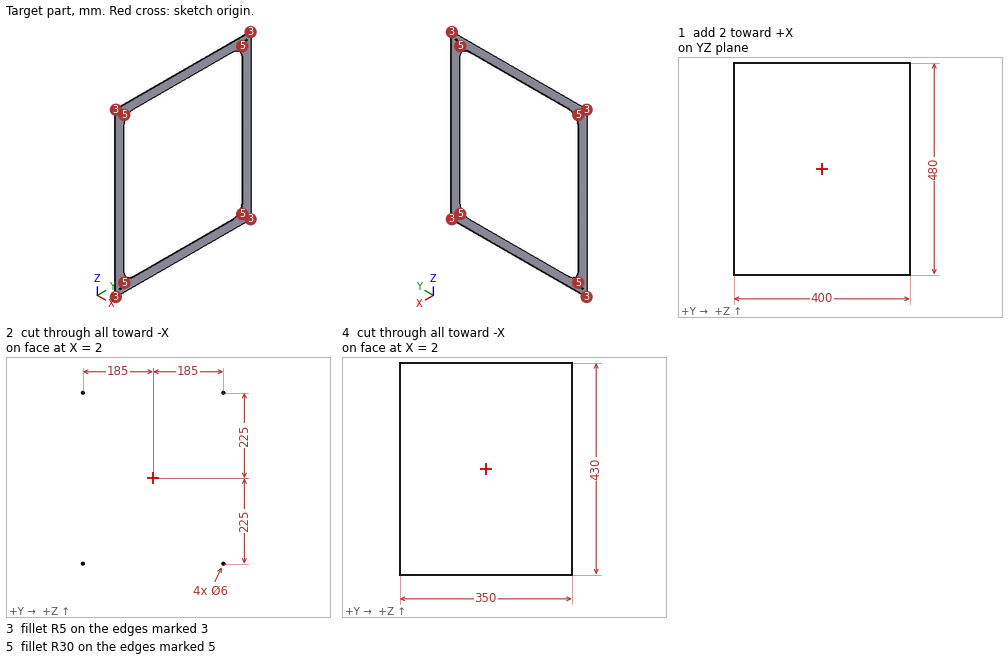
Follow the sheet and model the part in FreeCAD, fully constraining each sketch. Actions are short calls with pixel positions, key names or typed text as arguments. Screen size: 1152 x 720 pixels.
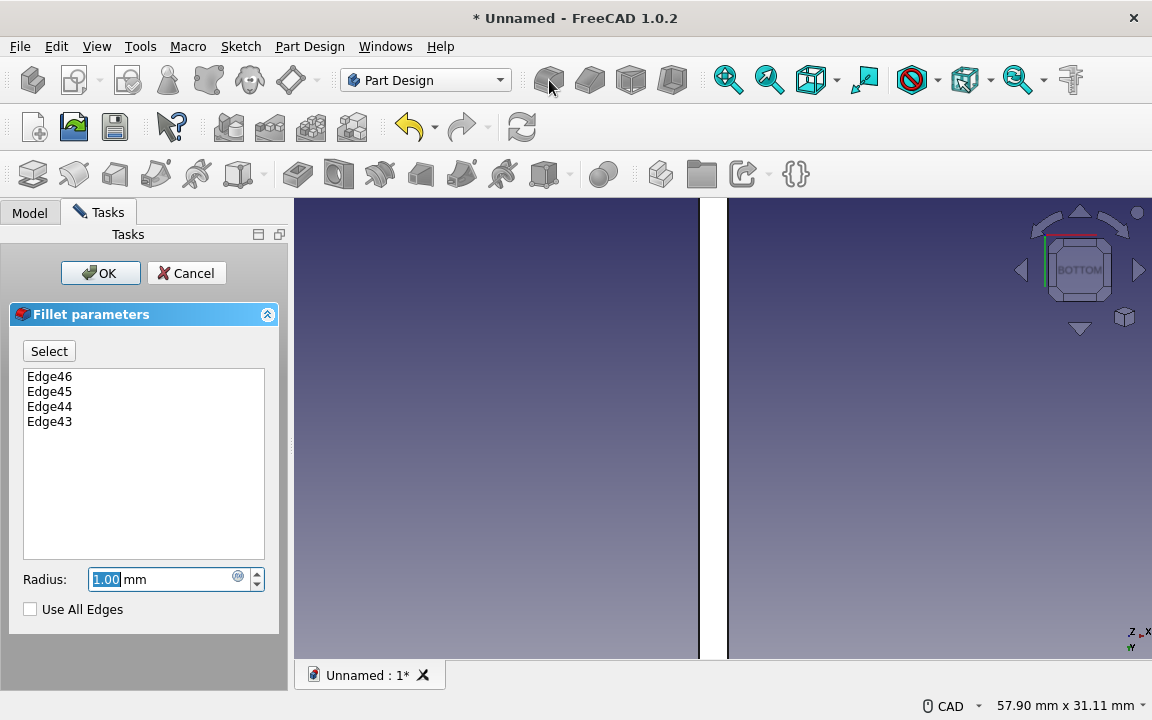
text(30)
key(Tab)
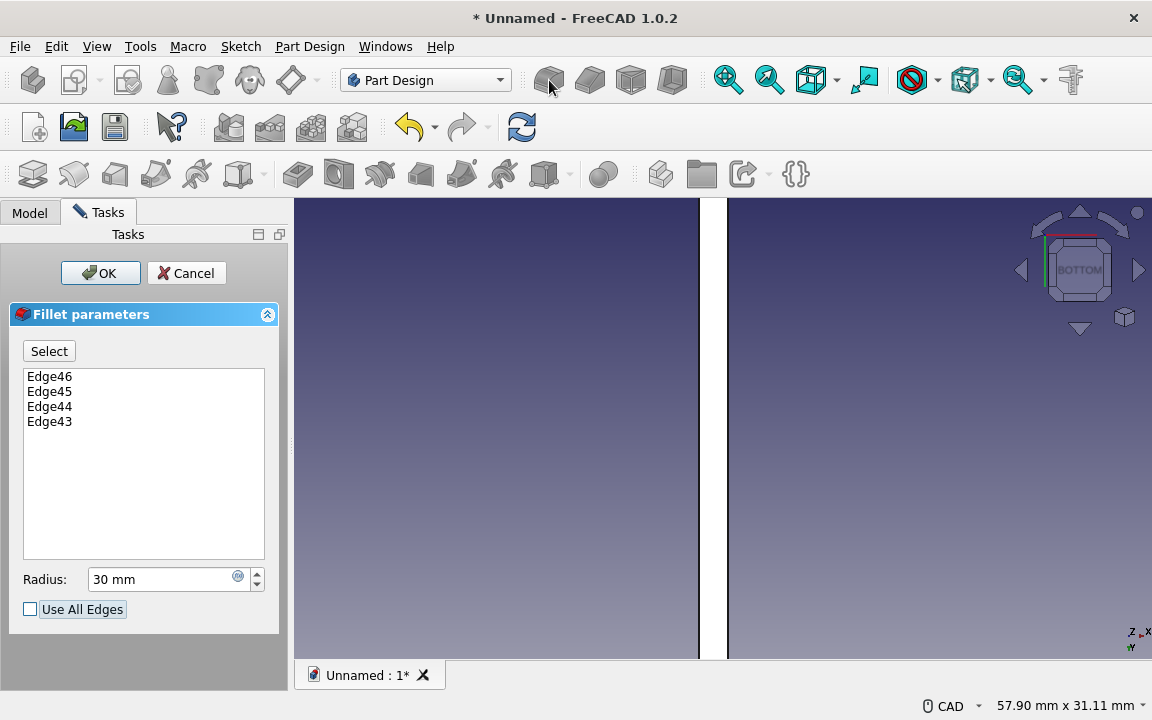
click(101, 273)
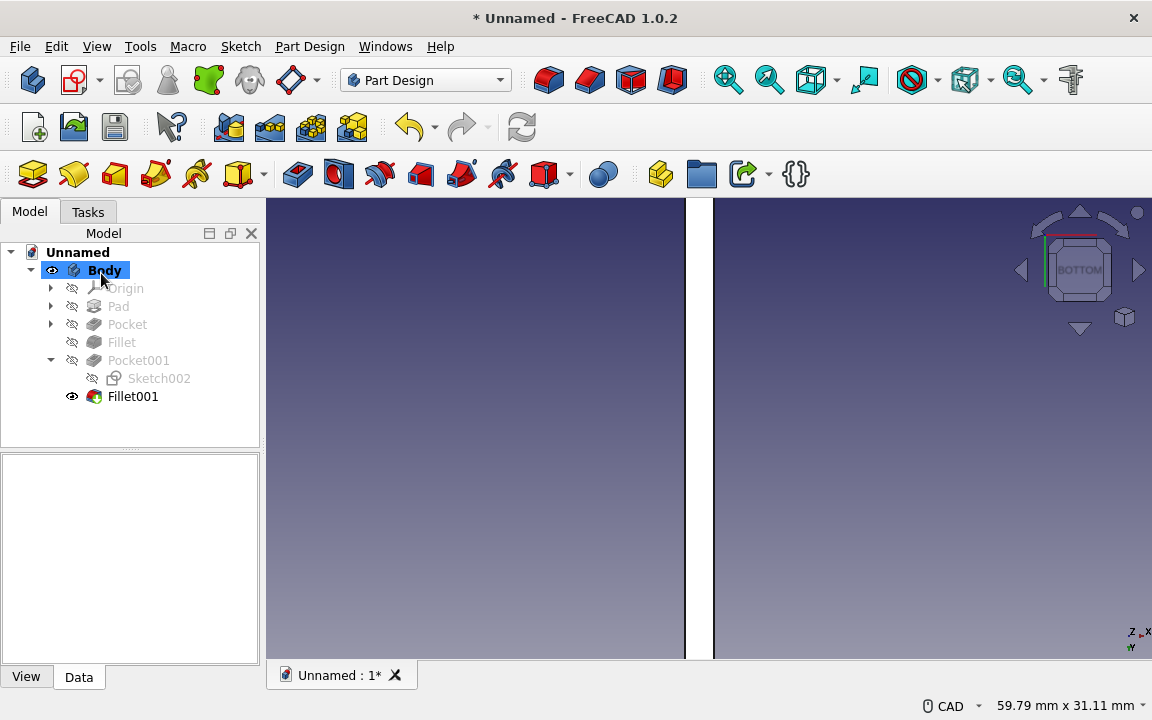
key(0)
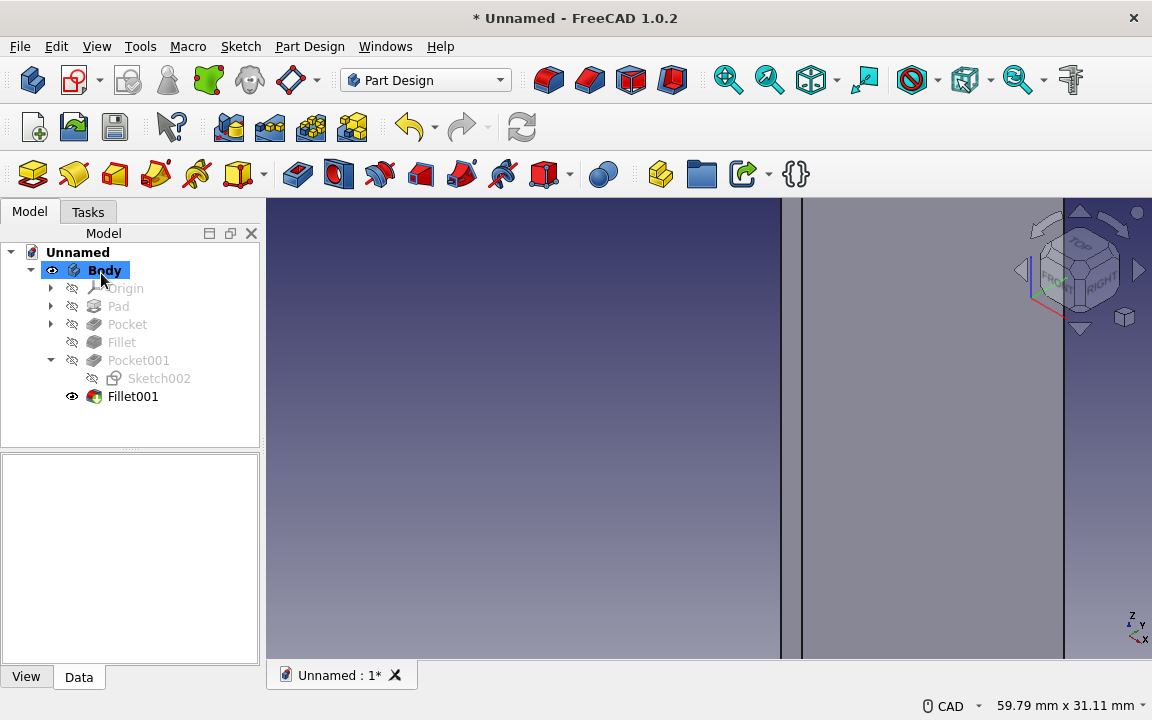
click(729, 80)